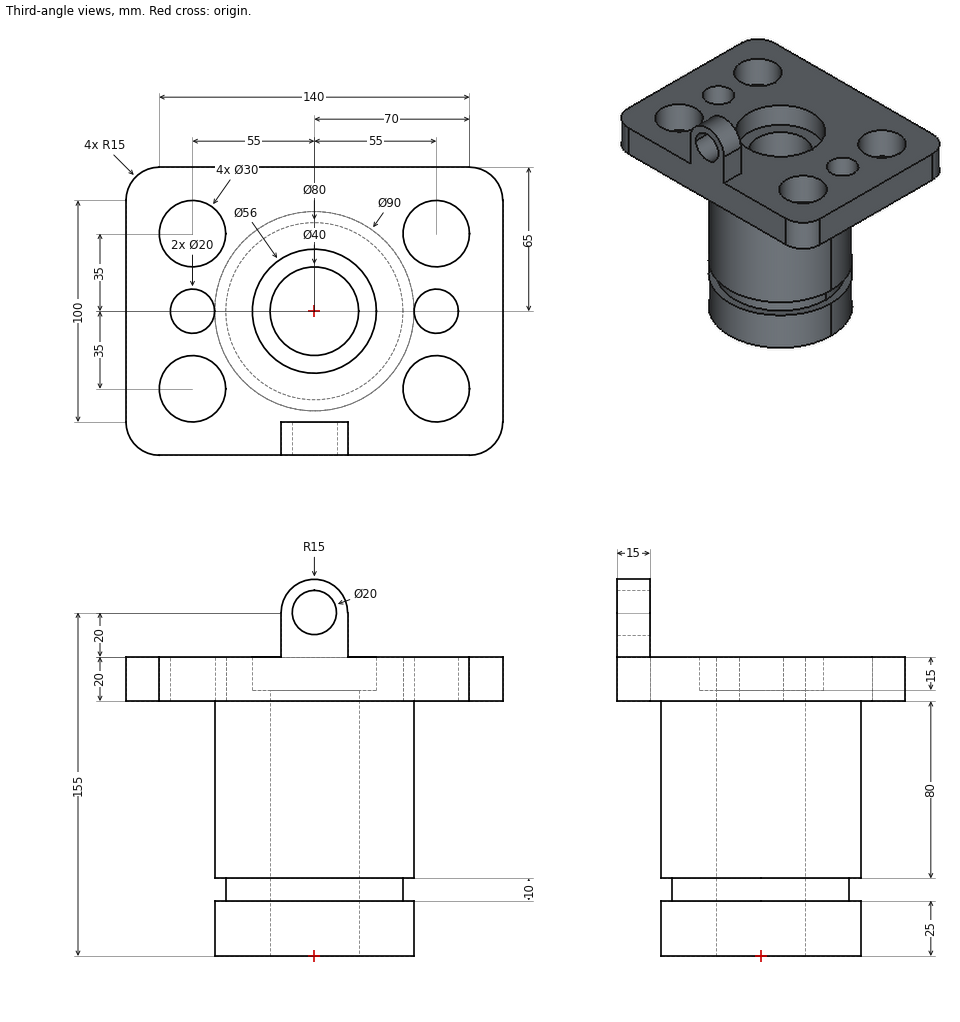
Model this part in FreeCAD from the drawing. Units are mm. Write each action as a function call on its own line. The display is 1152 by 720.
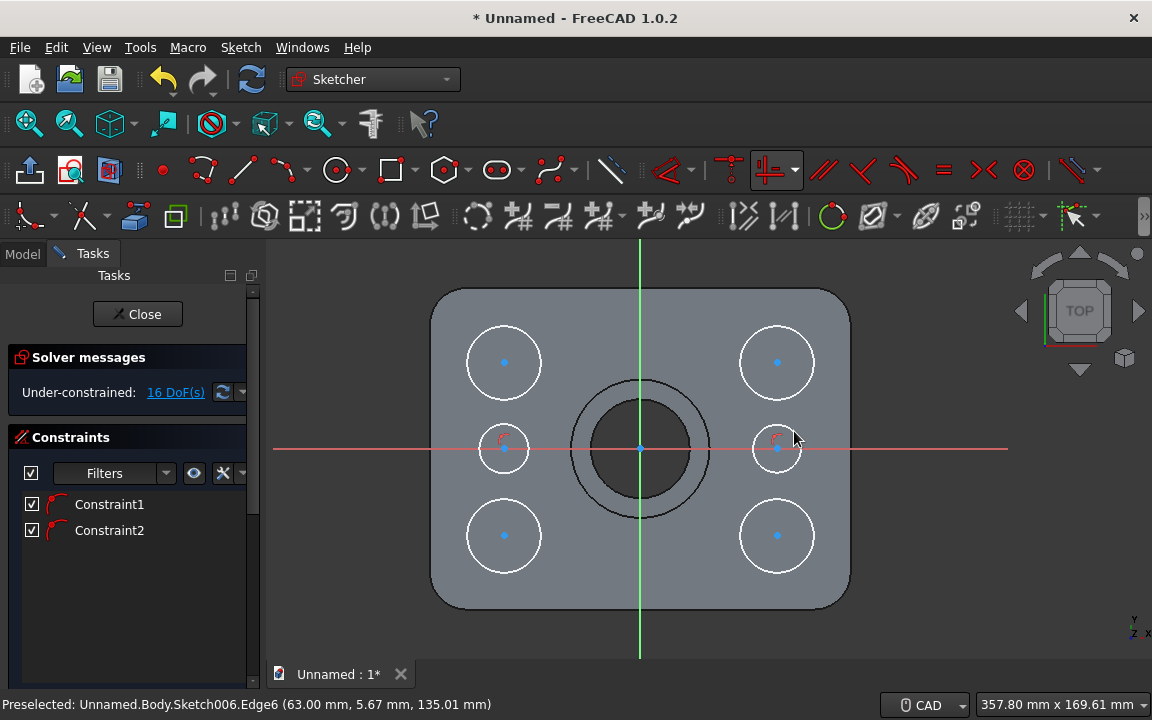
click(530, 337)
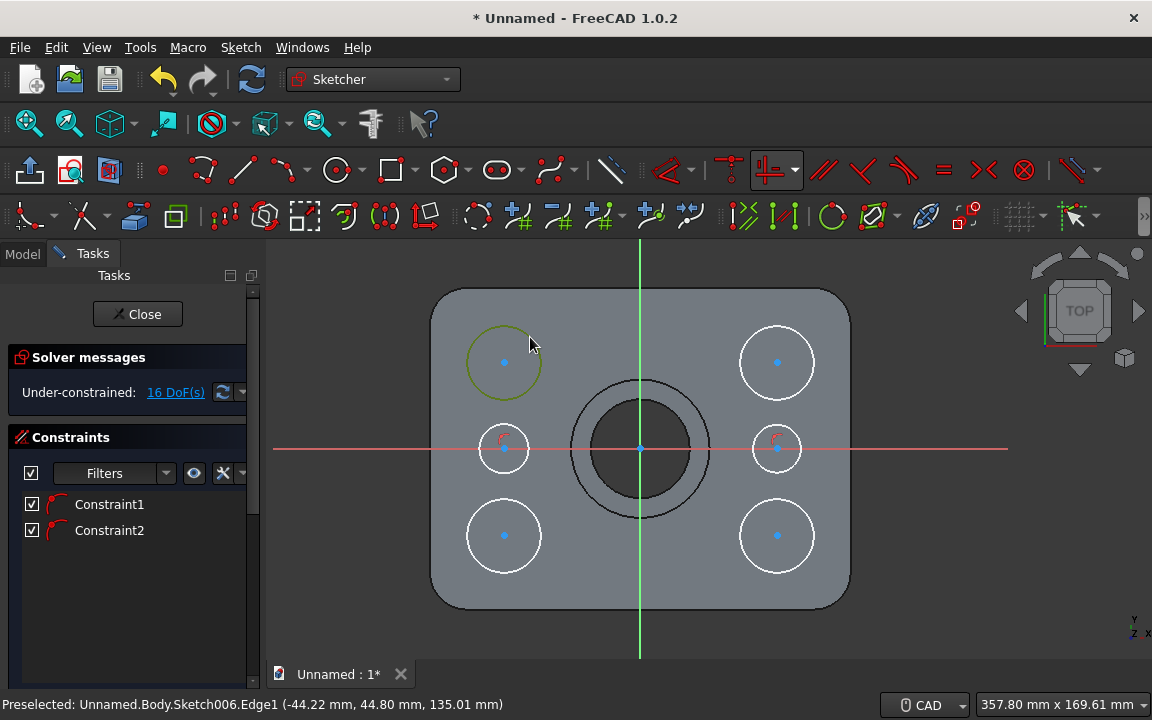
click(803, 337)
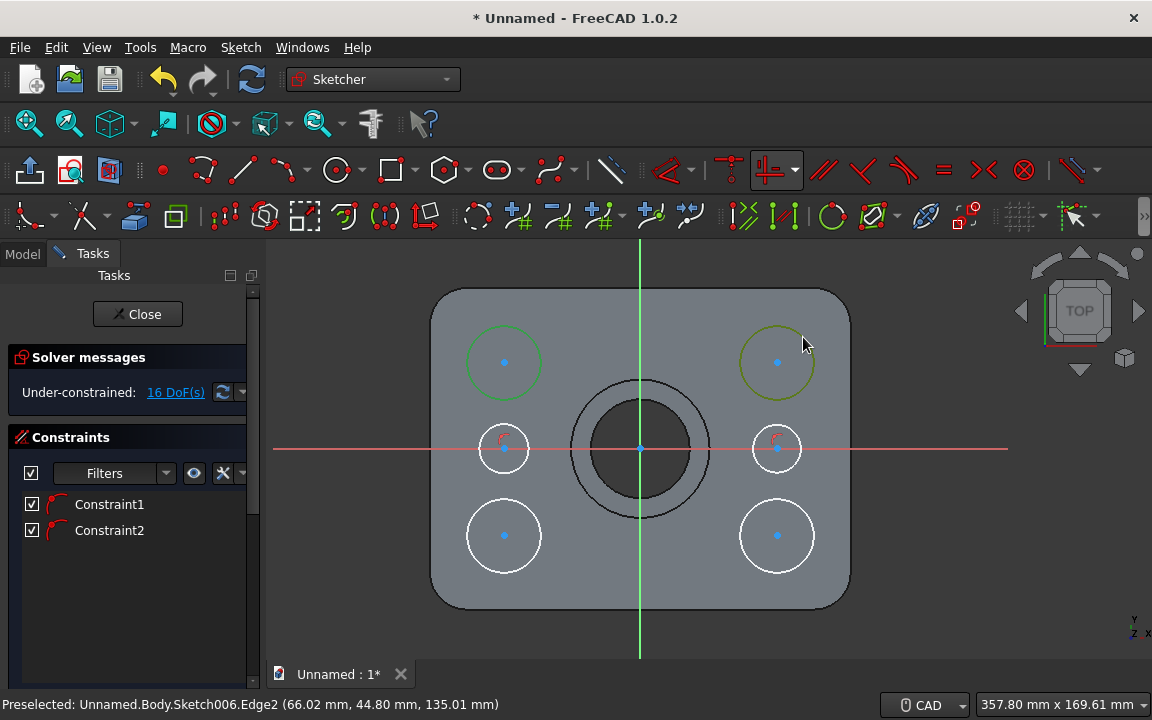
click(530, 510)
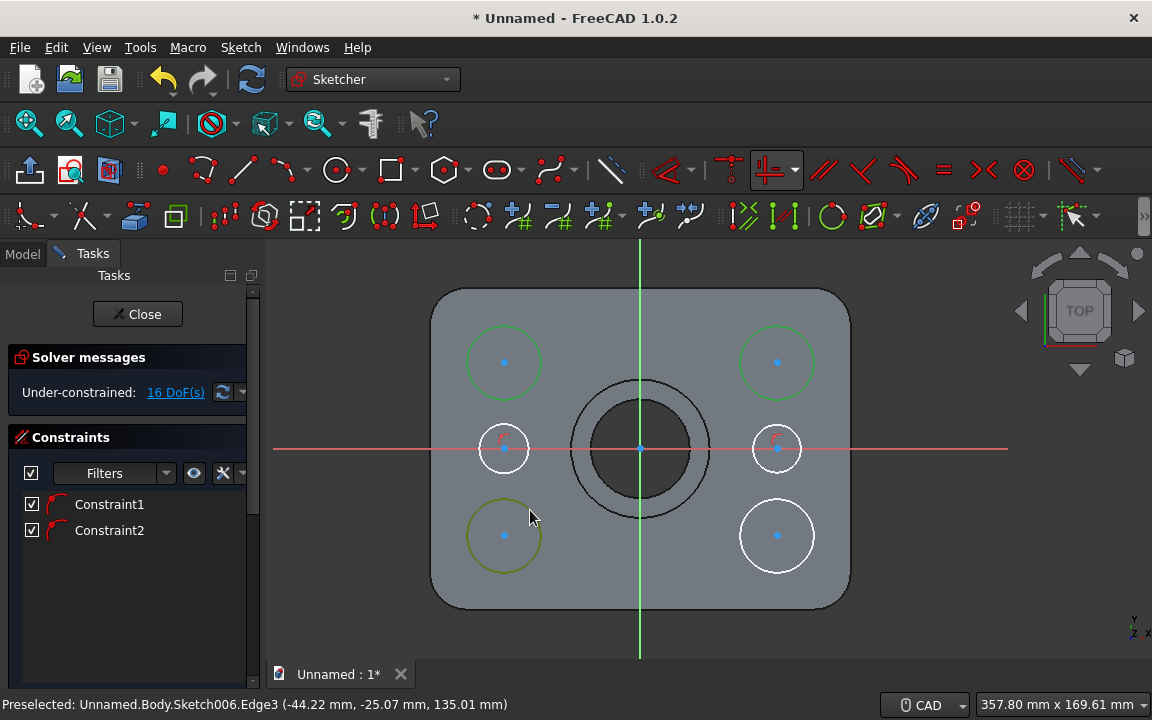
click(803, 510)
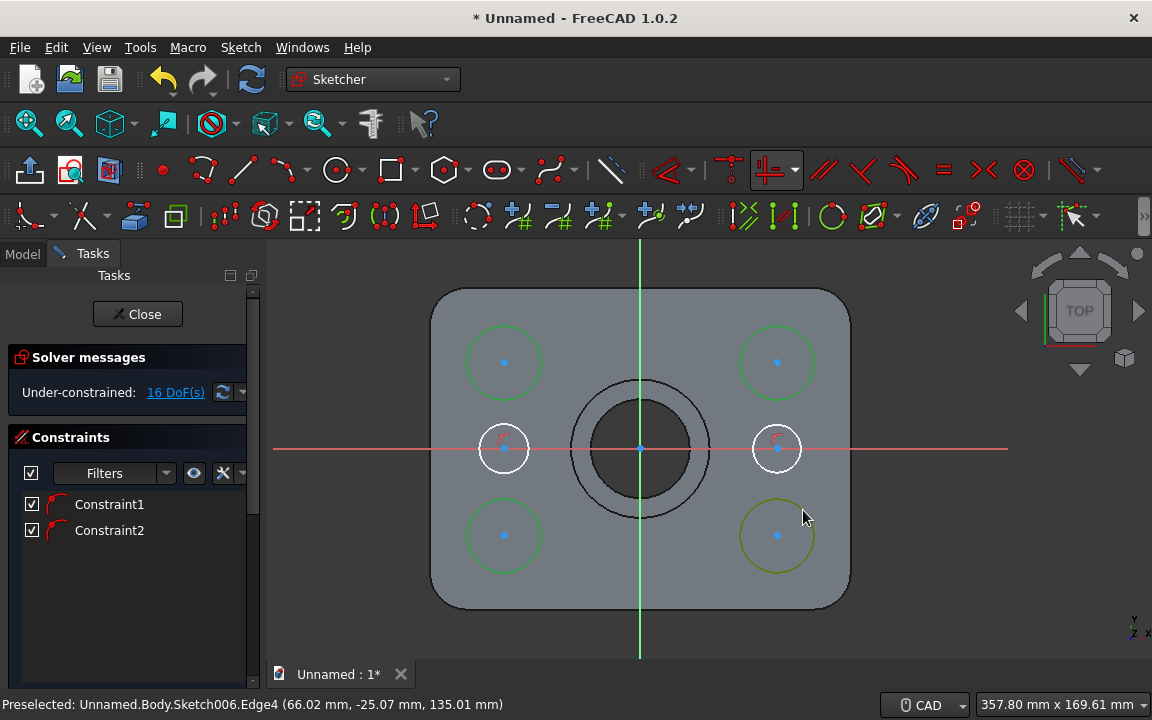
click(944, 170)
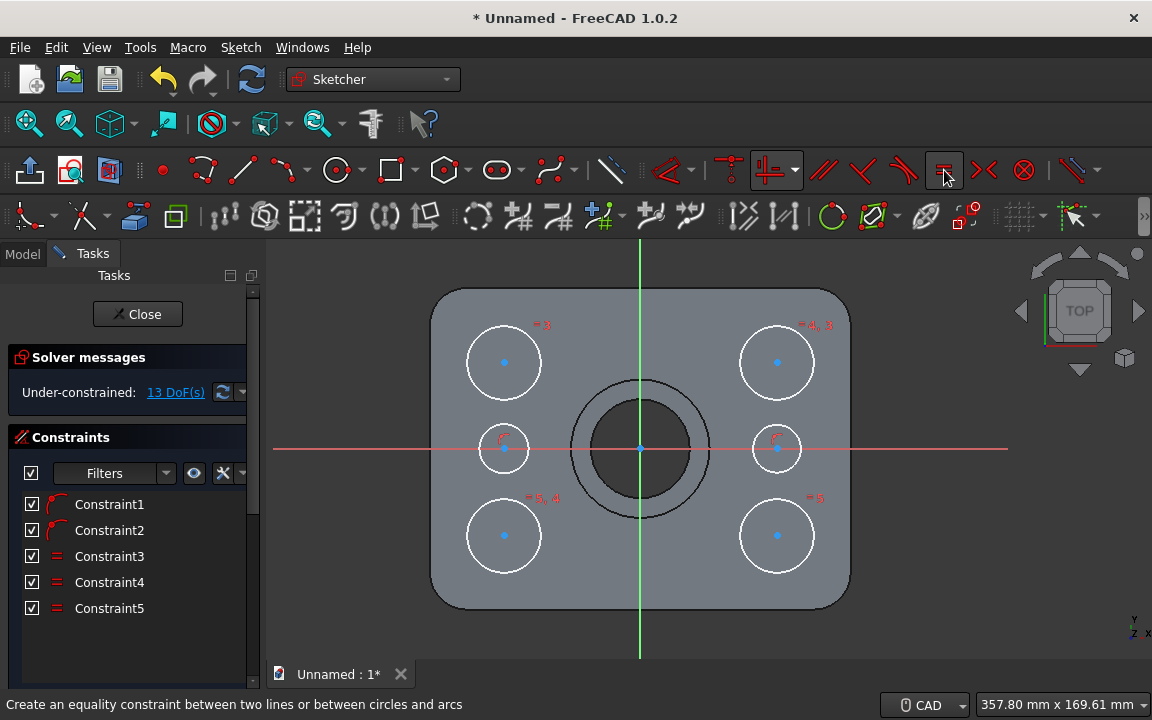
click(521, 431)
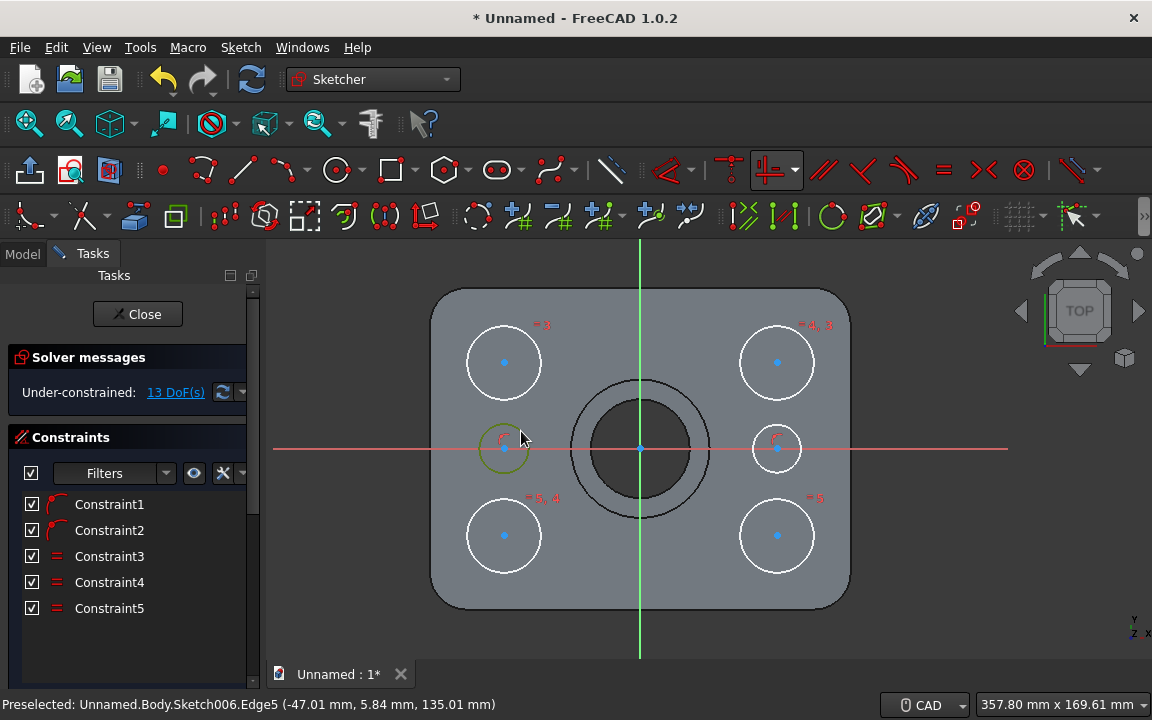
click(794, 432)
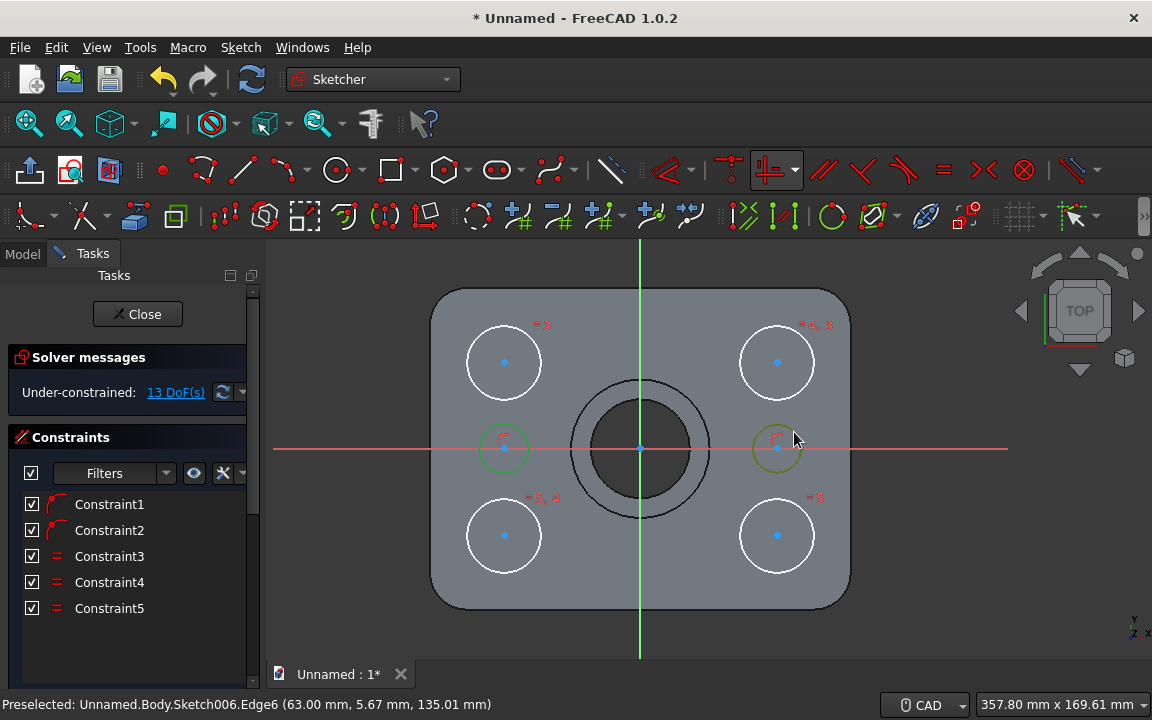
click(944, 170)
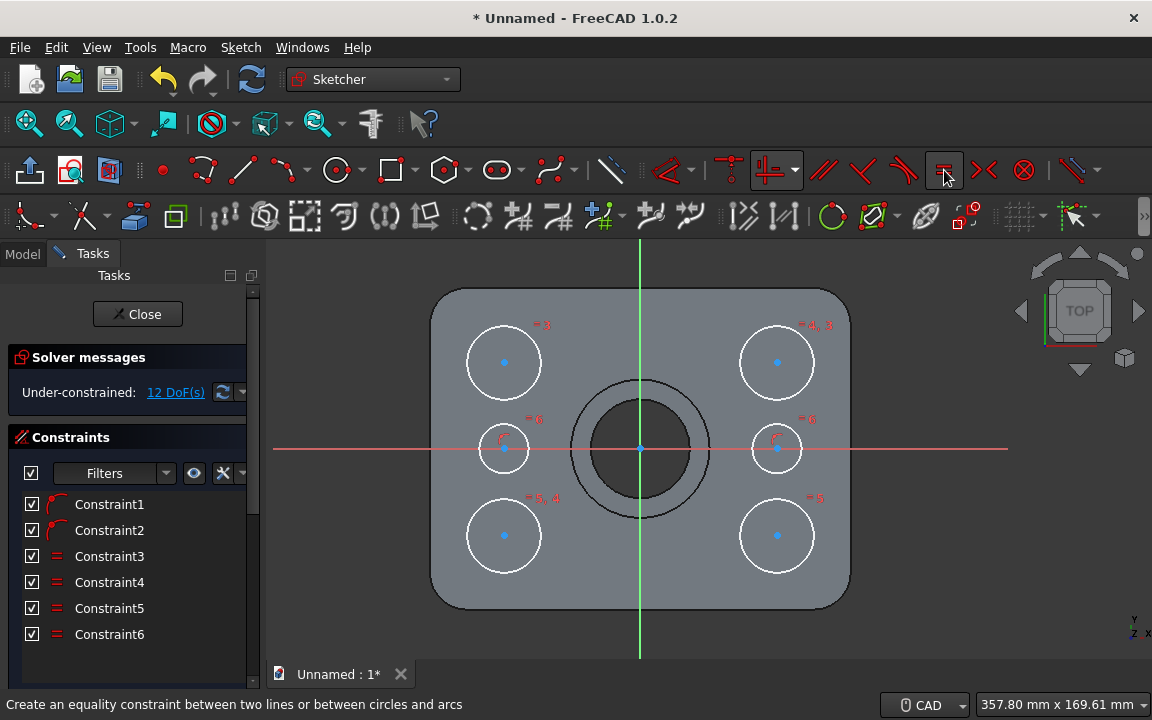
click(666, 170)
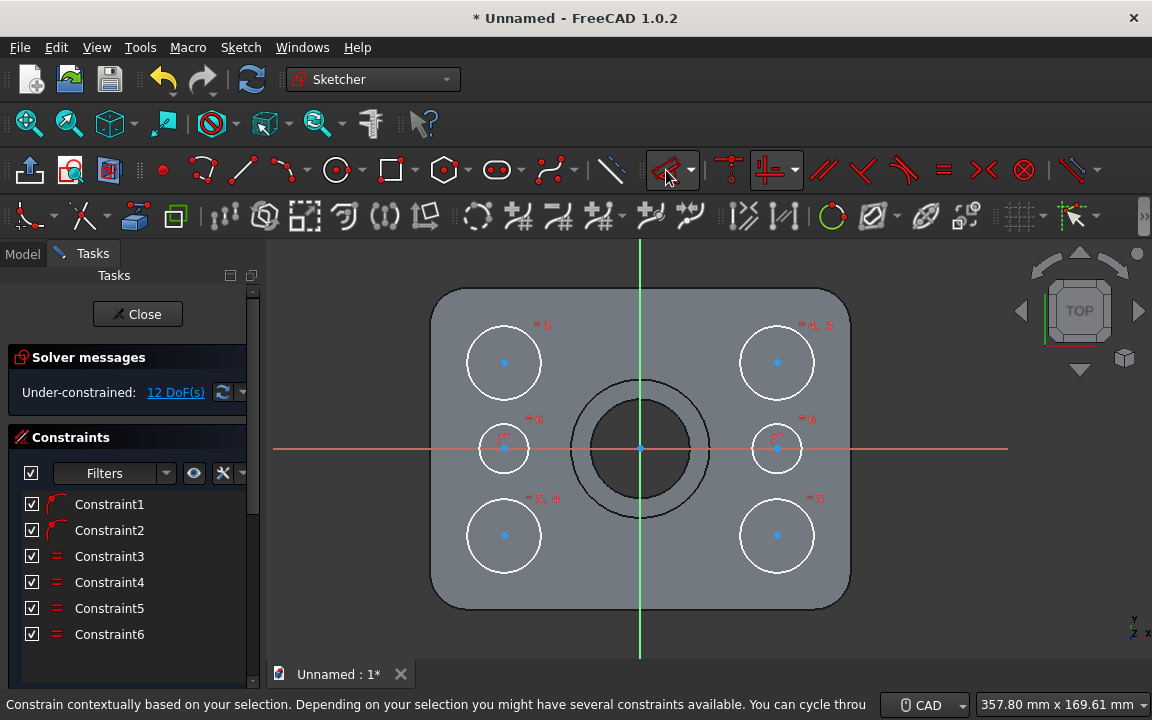
click(530, 337)
click(553, 314)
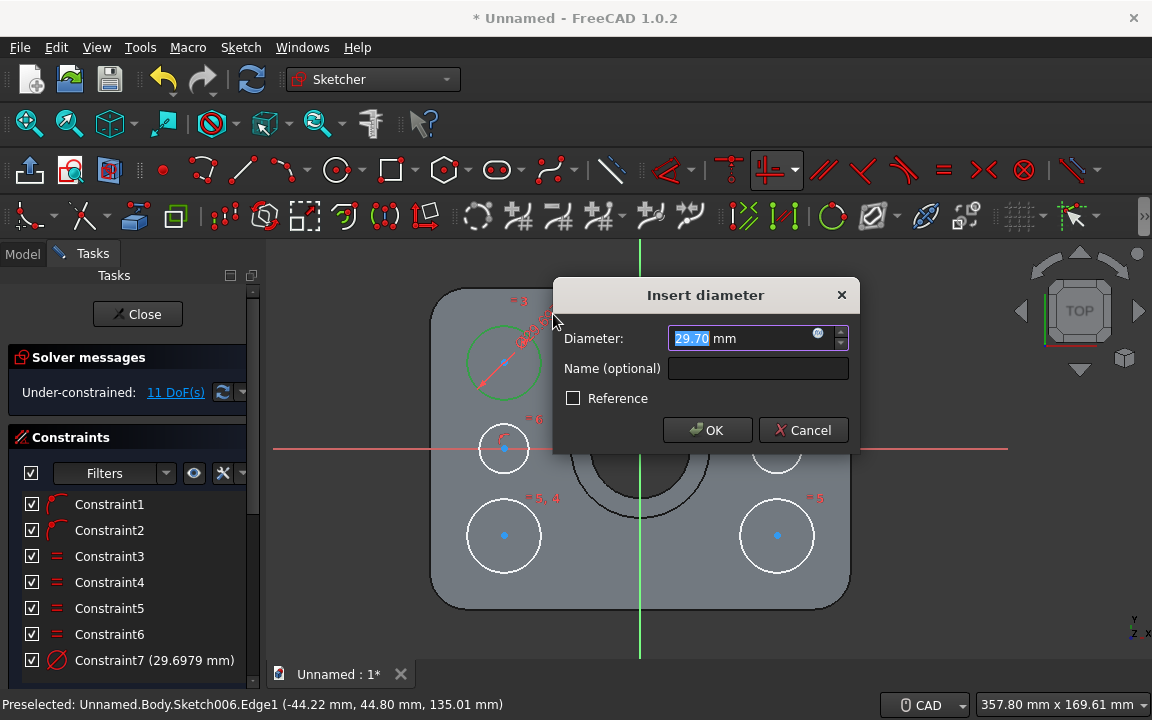
text(30)
key(Return)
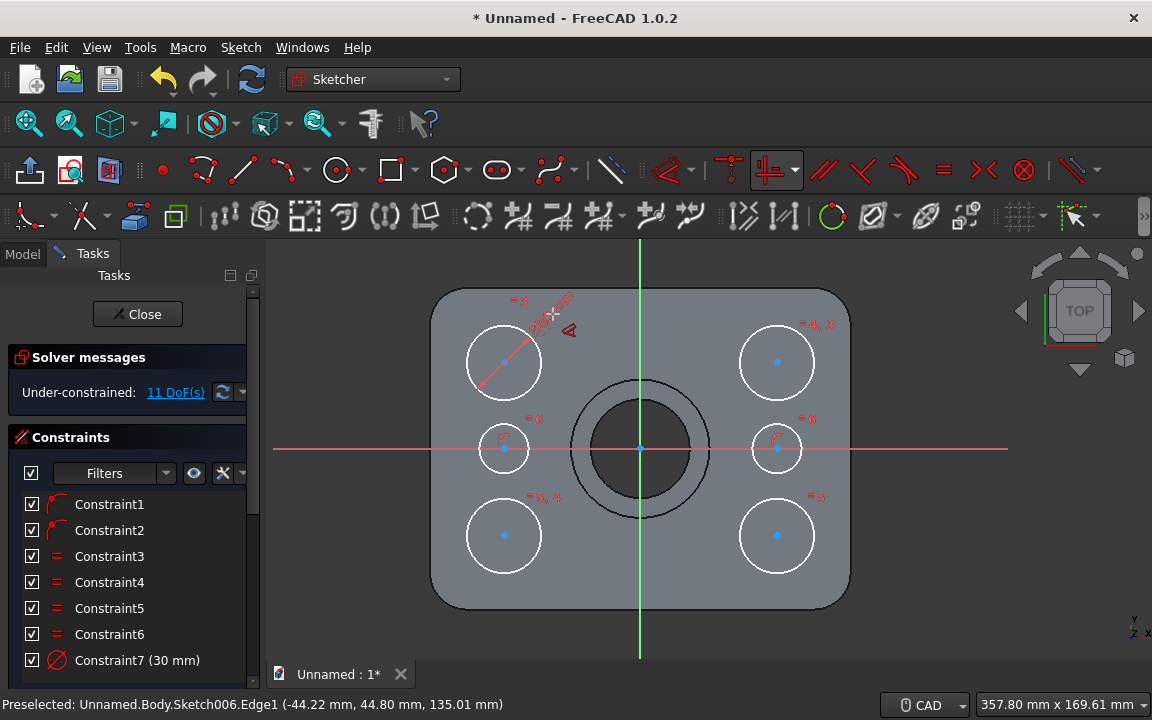
click(521, 431)
click(543, 408)